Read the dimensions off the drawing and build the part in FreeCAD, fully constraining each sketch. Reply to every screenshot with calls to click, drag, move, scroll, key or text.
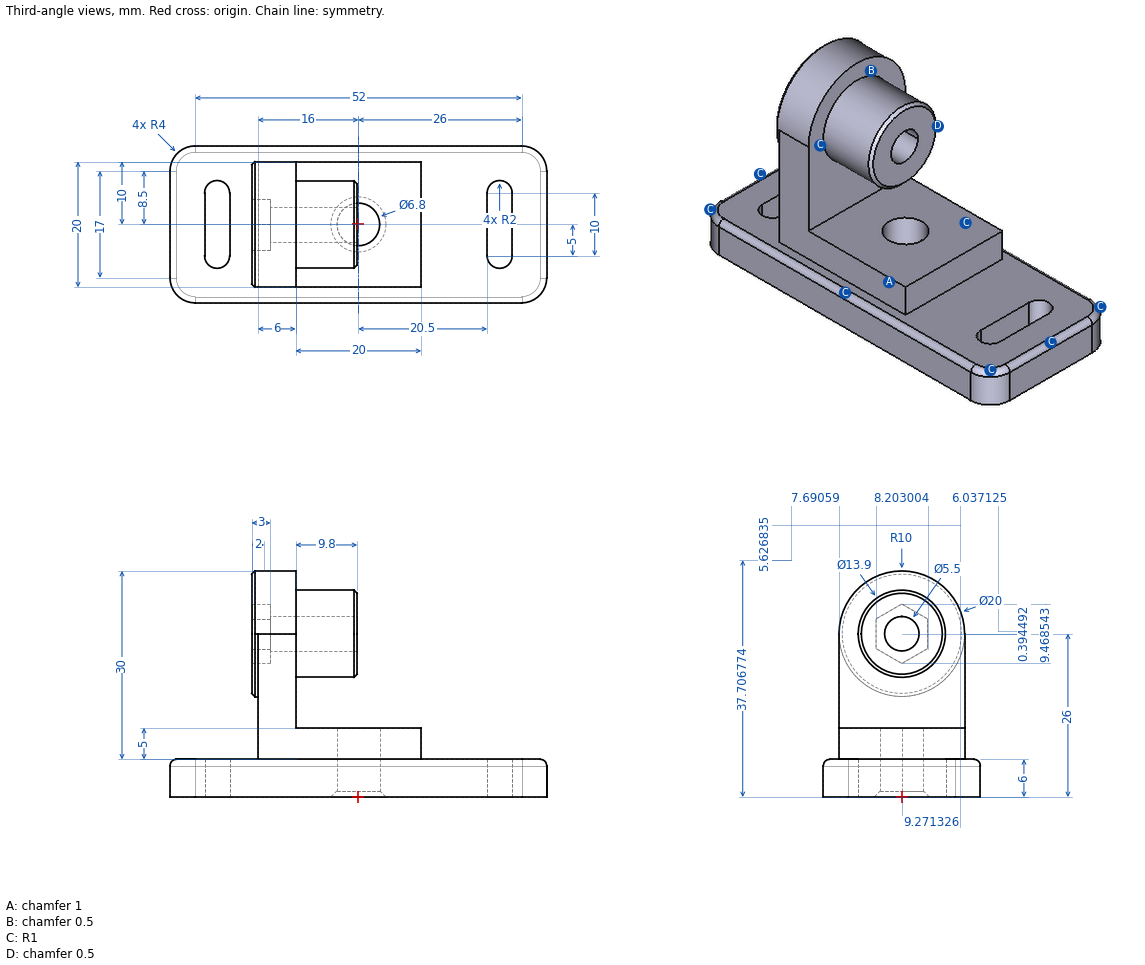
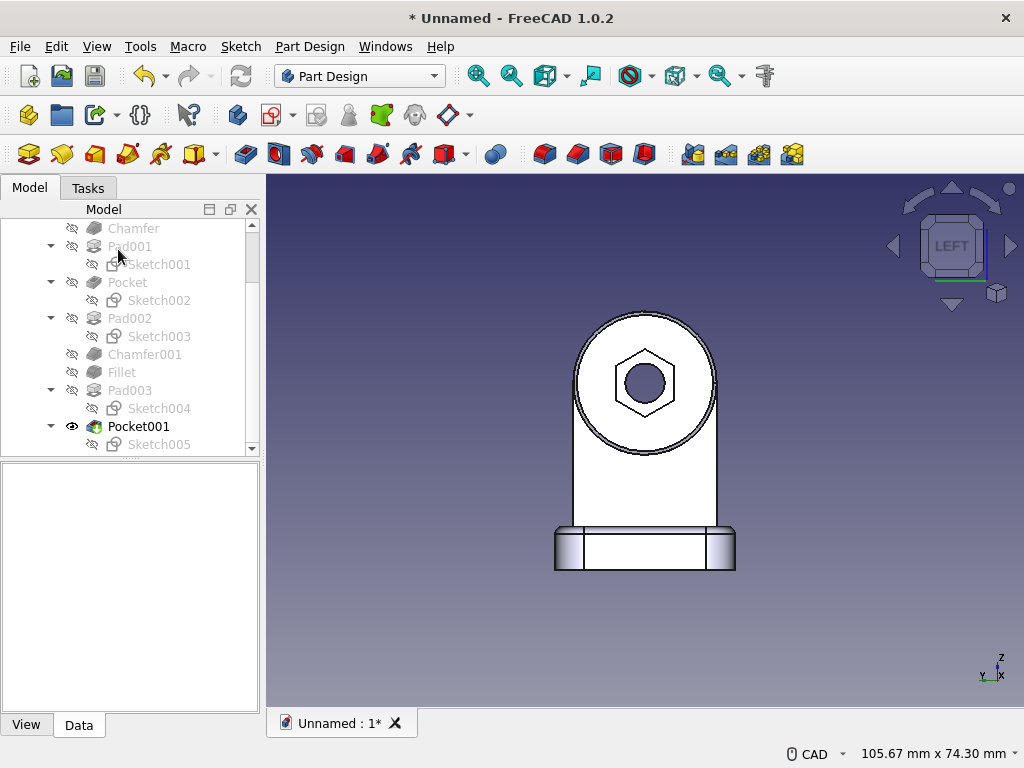
key(0)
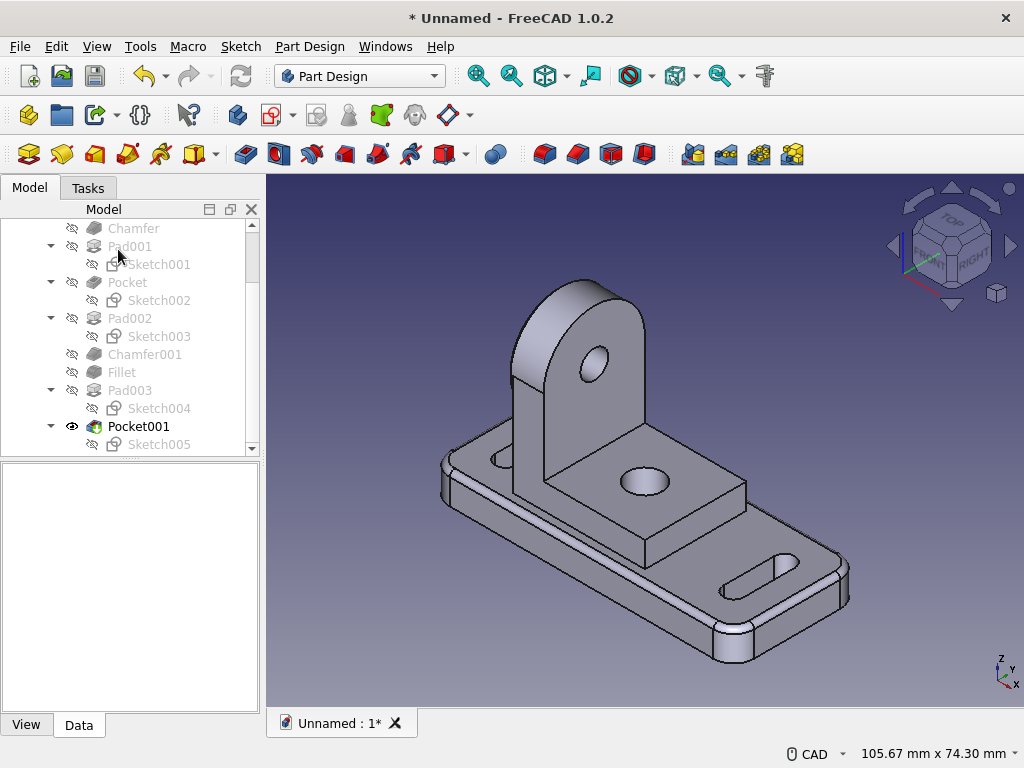
click(609, 411)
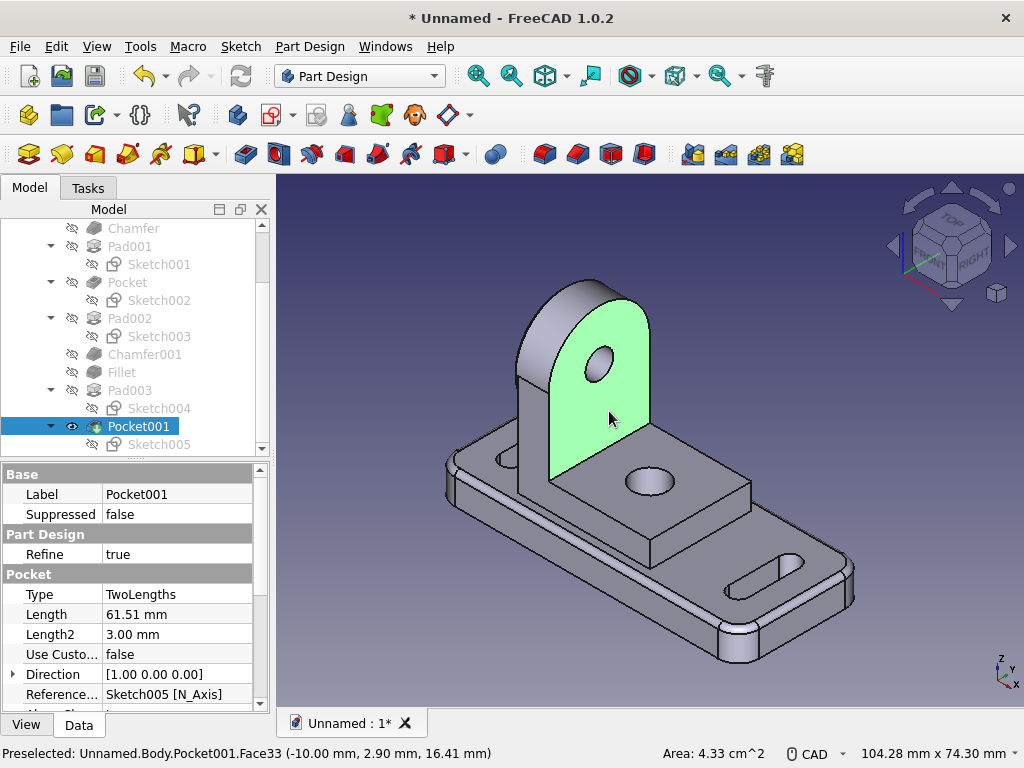
click(270, 116)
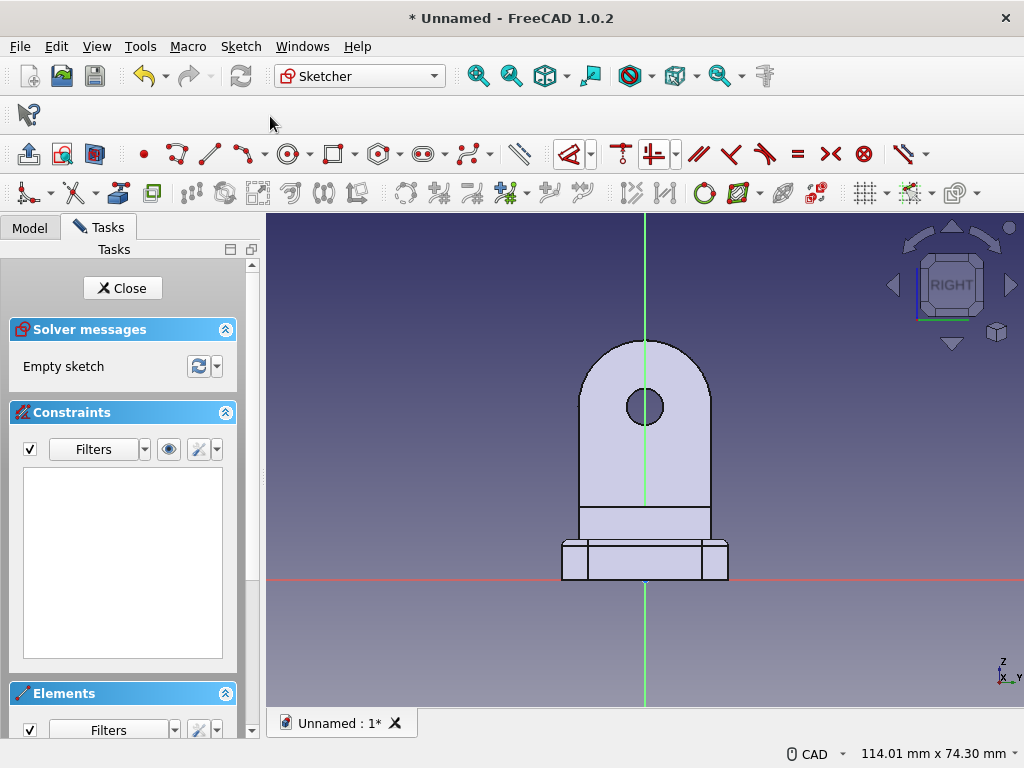
click(95, 154)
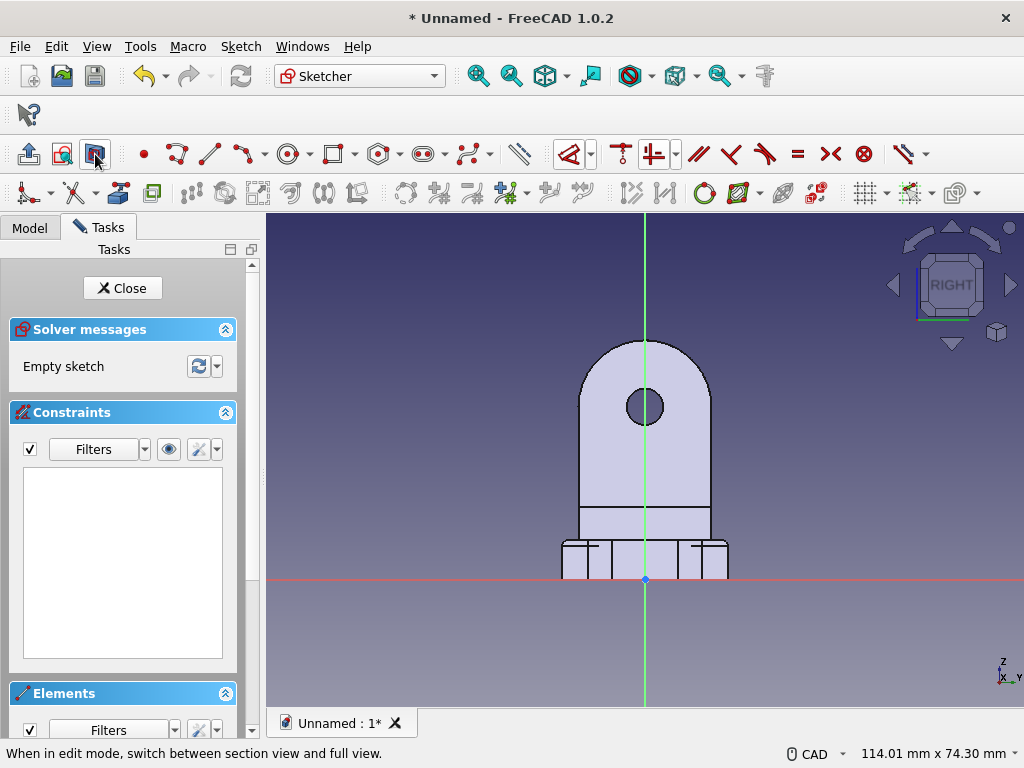
scroll(784, 491, up, 2)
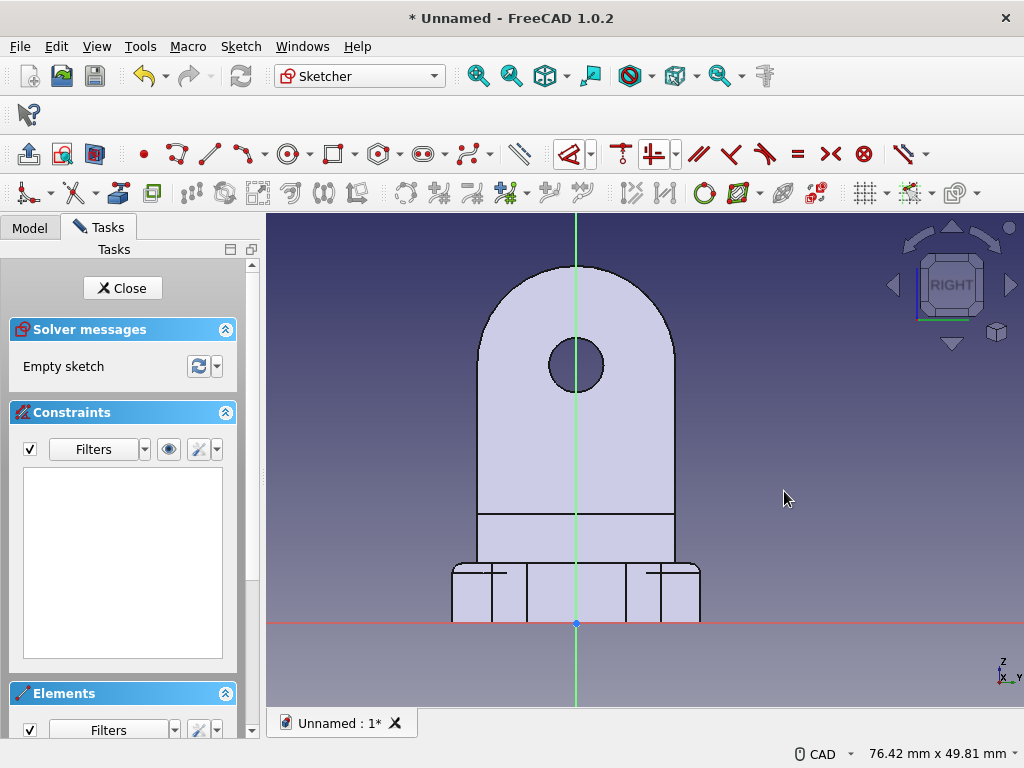
click(288, 154)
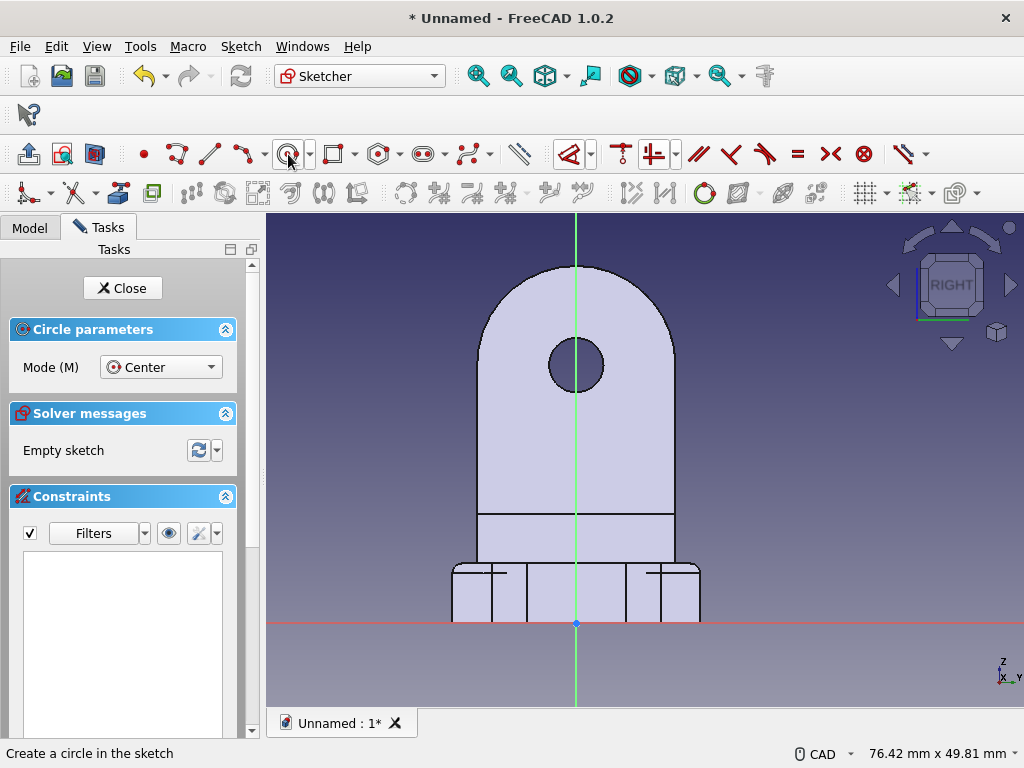
click(576, 365)
move(625, 316)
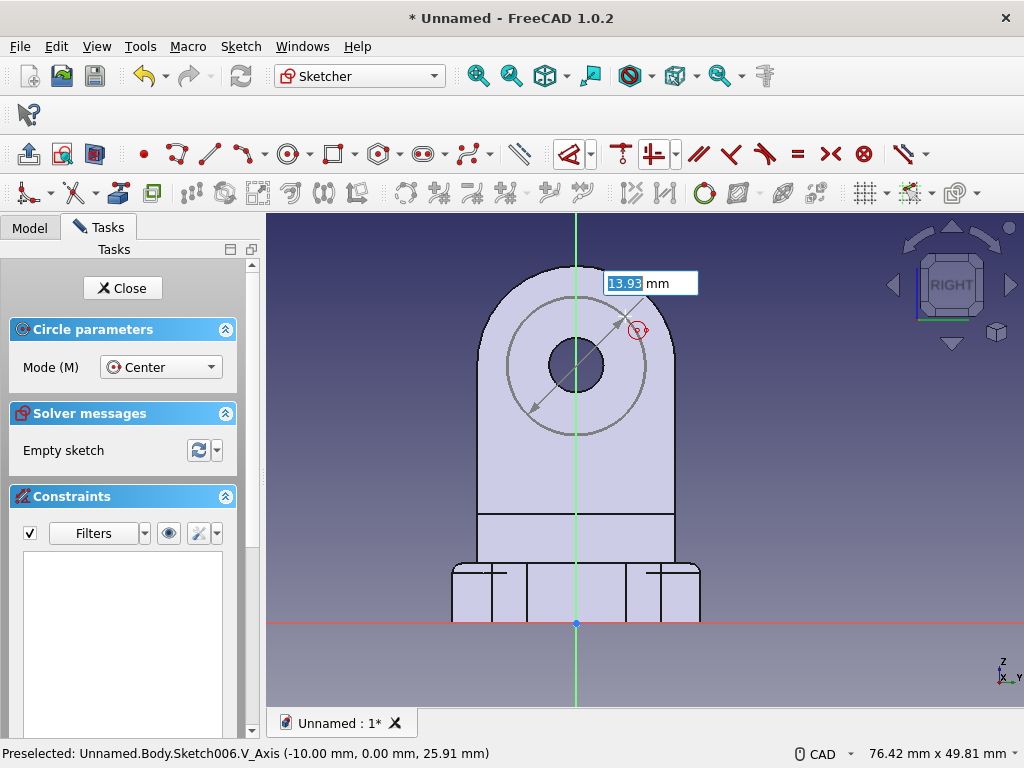
text(13.9)
key(Return)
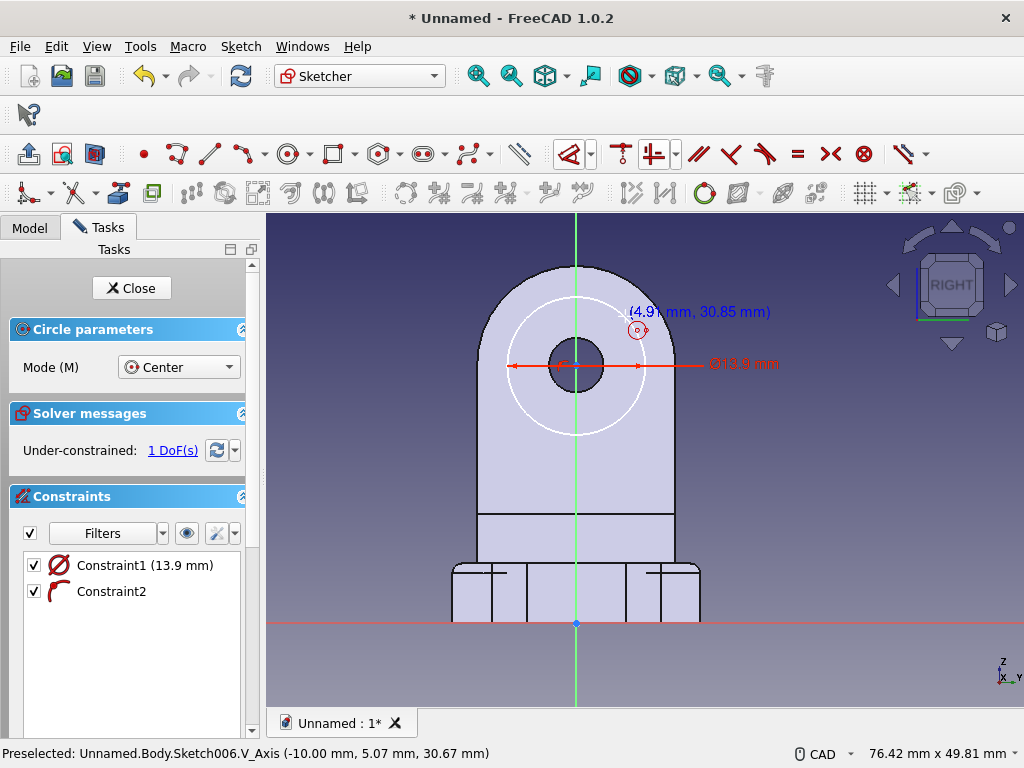
click(576, 366)
move(596, 346)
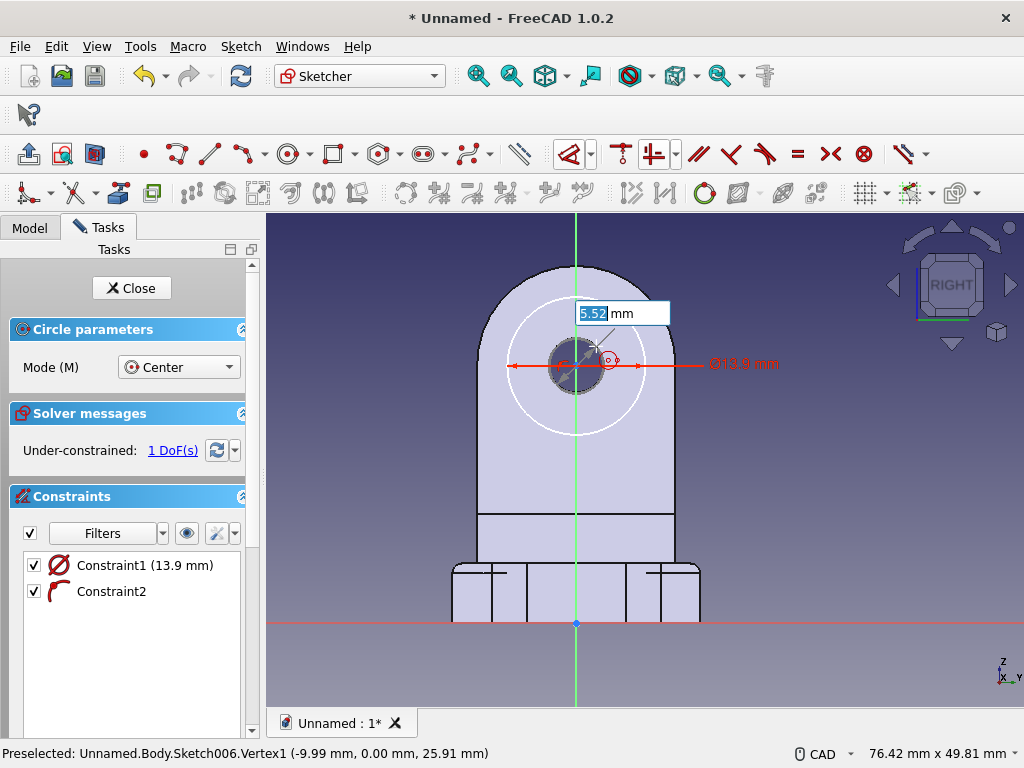
text(5.5)
key(Return)
key(Escape)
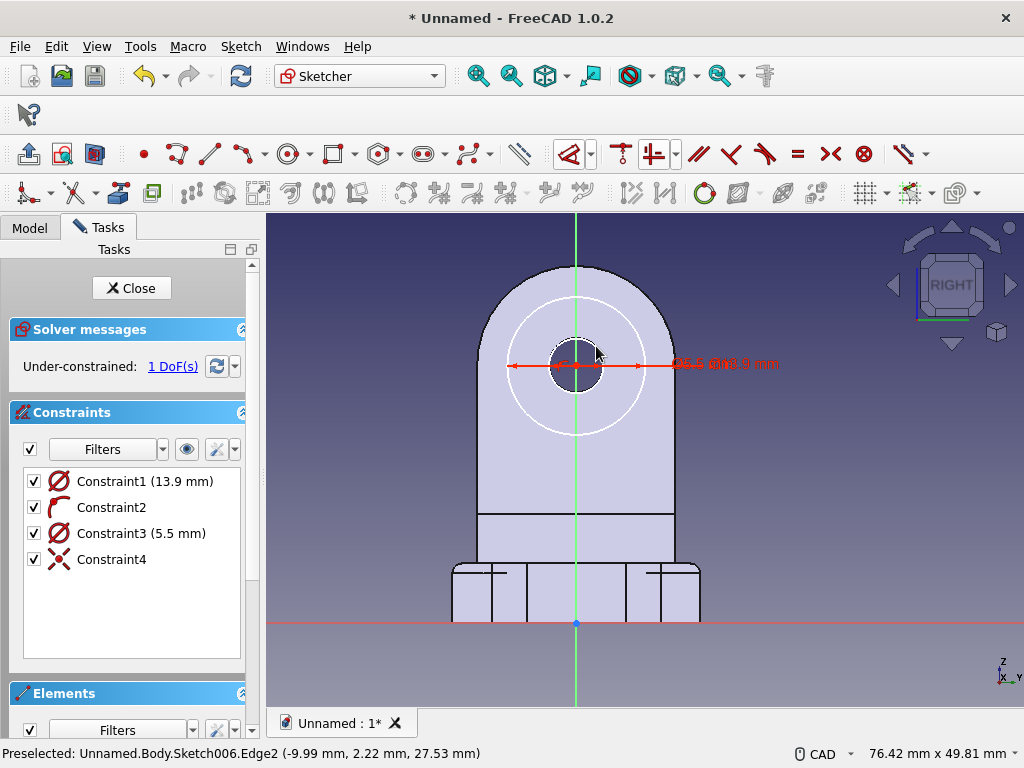
click(576, 366)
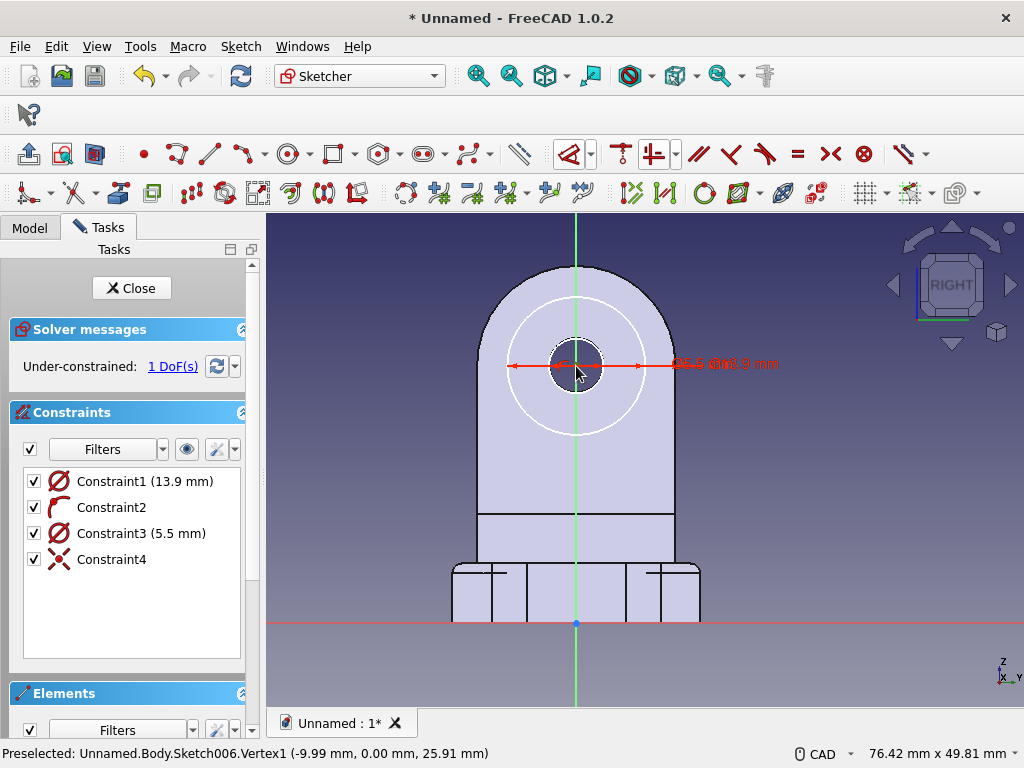
key(i)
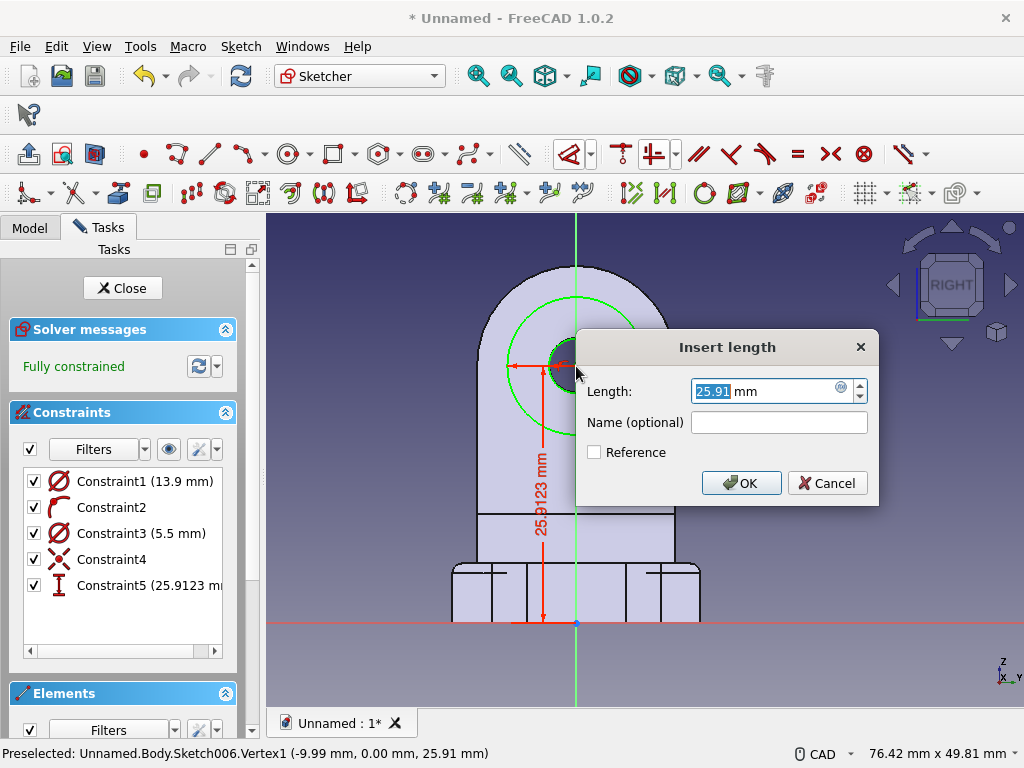
text(26)
key(Return)